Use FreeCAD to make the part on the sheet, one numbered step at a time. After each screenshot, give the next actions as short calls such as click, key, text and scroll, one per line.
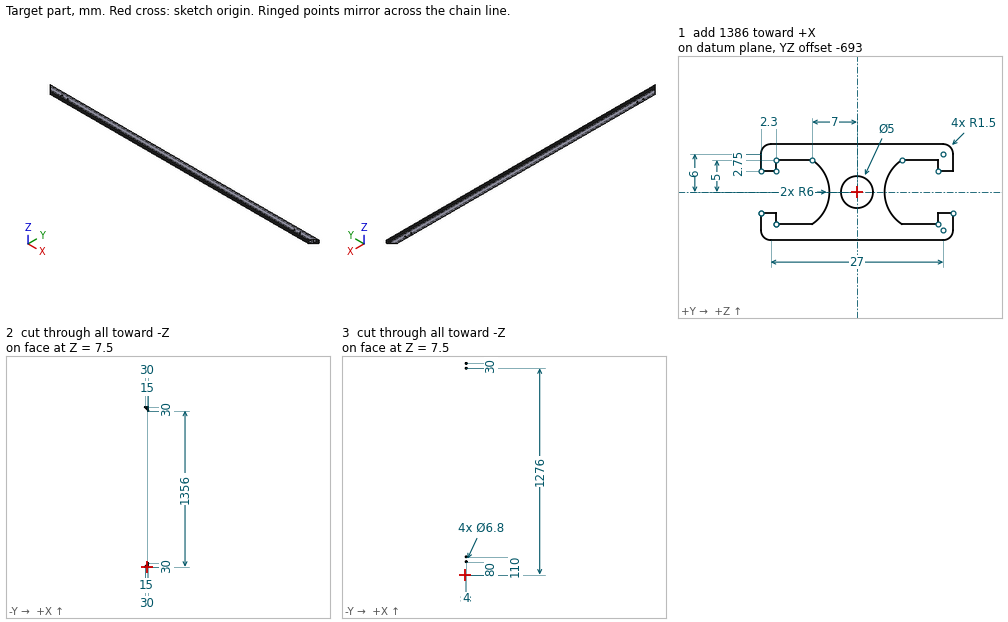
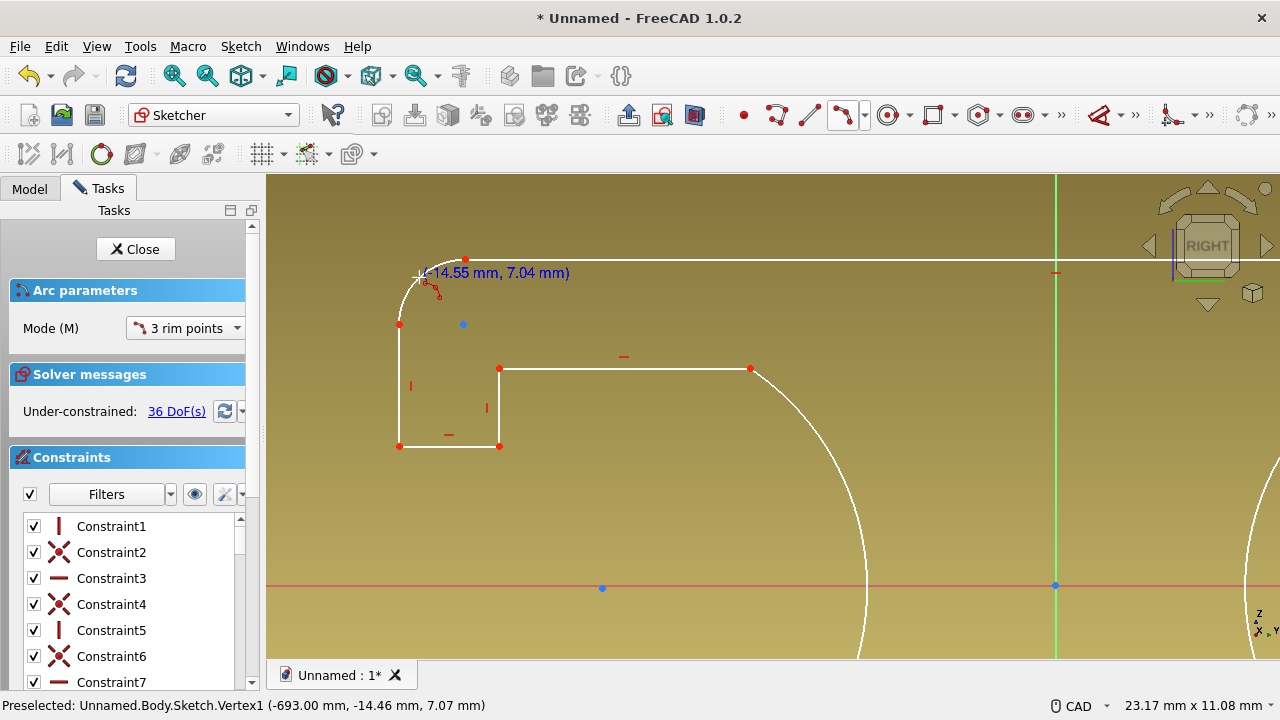
click(888, 116)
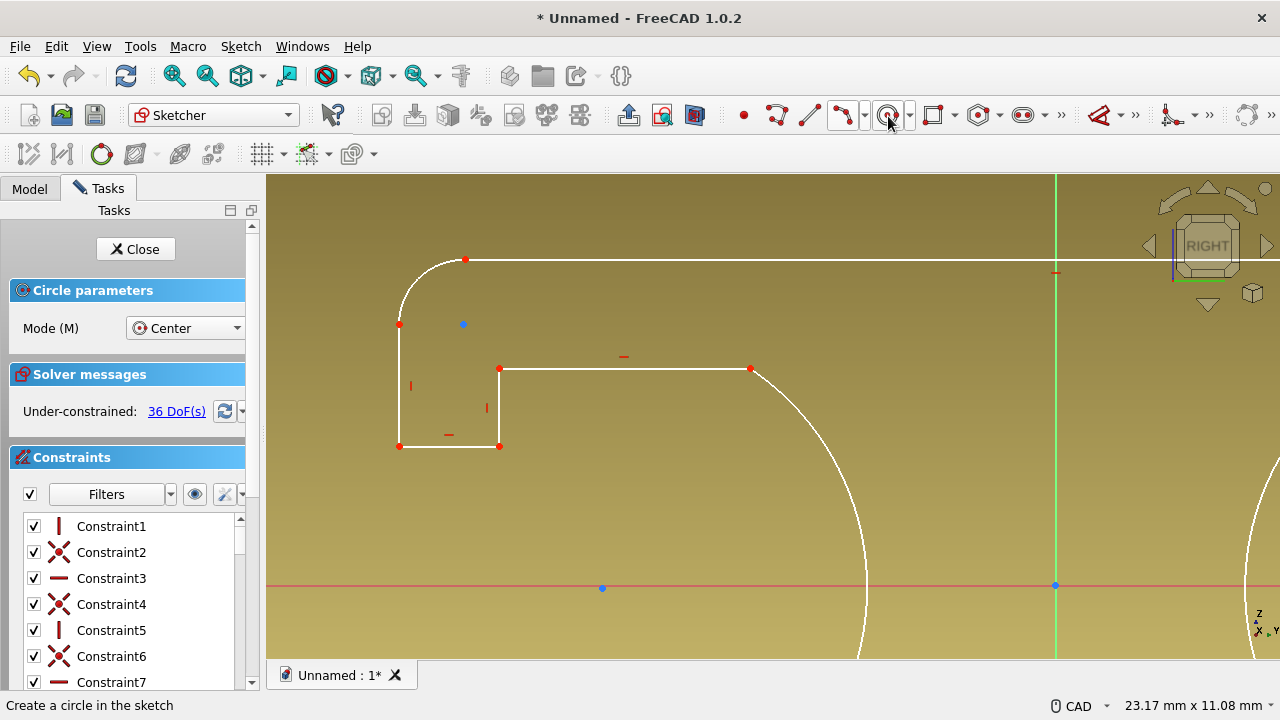
click(1056, 586)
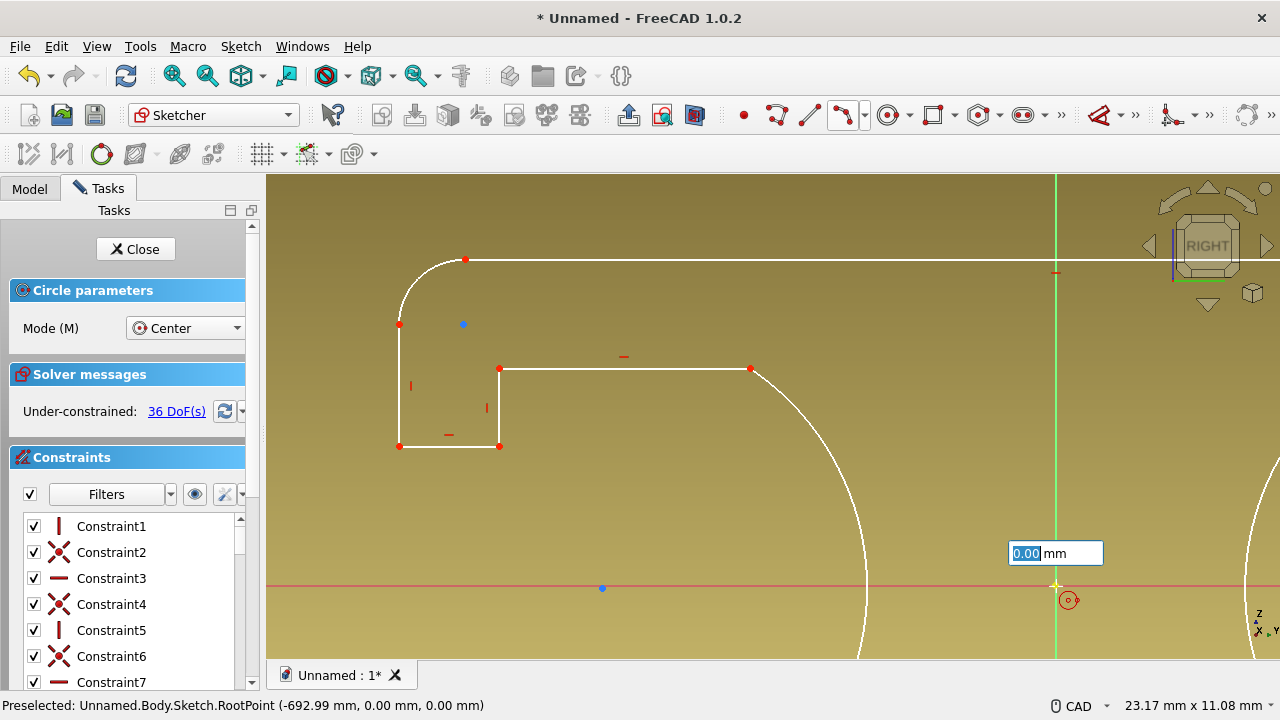
scroll(418, 278, down, 4)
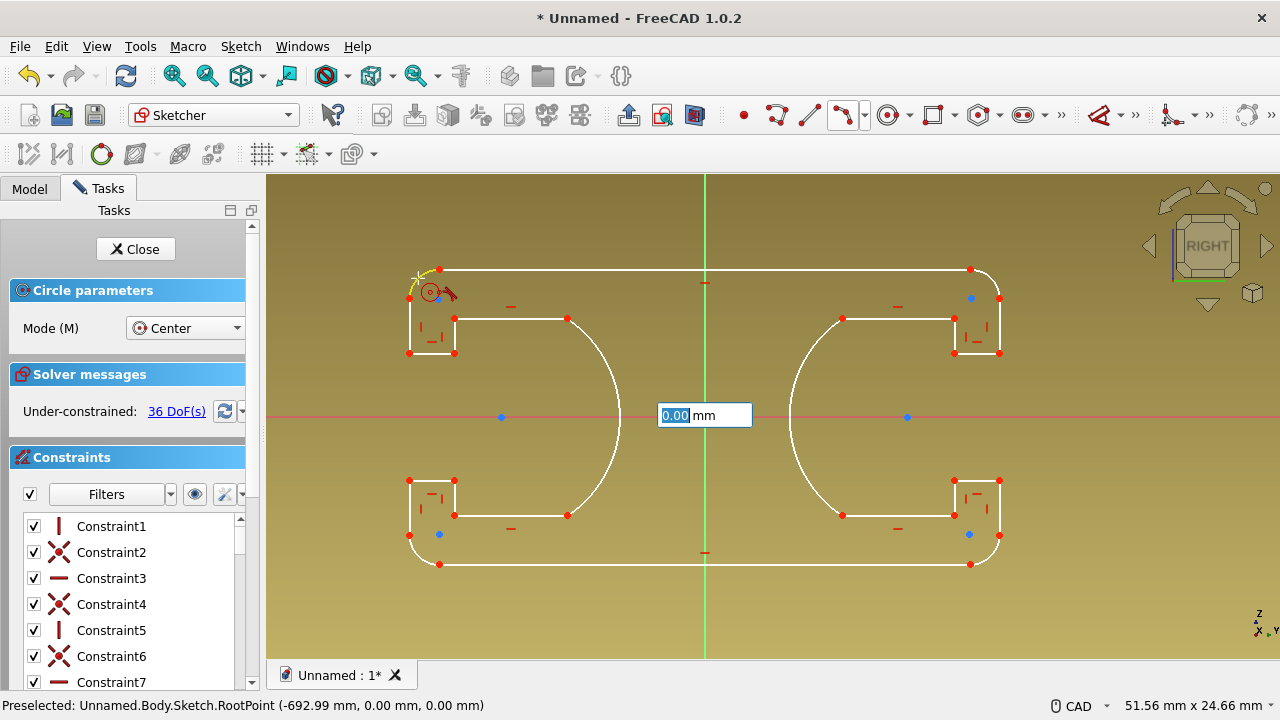
click(740, 382)
key(Escape)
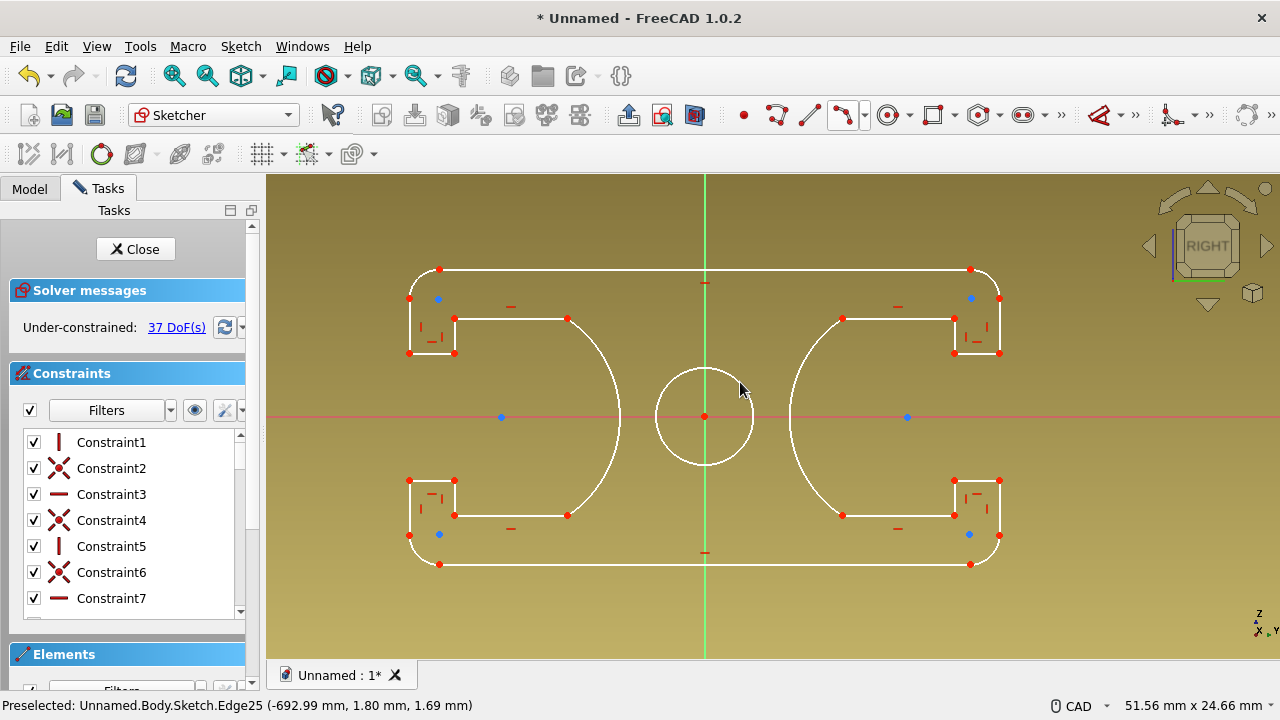
click(410, 315)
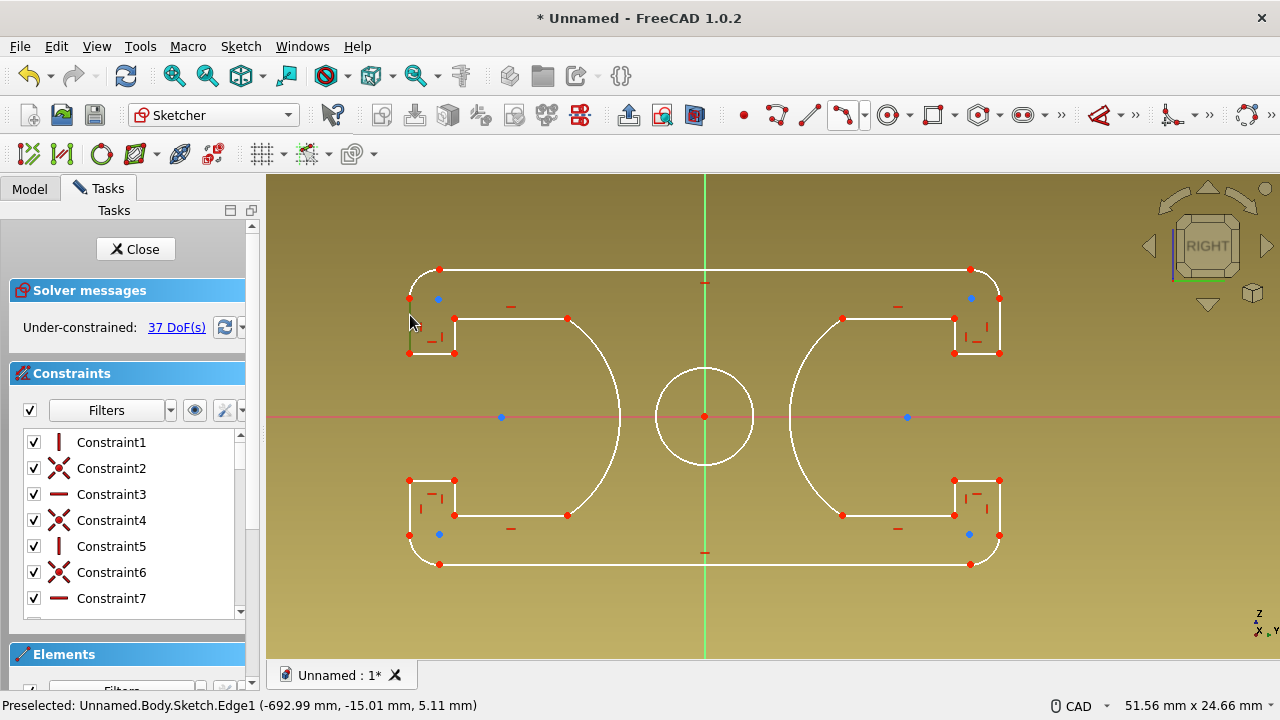
click(426, 273)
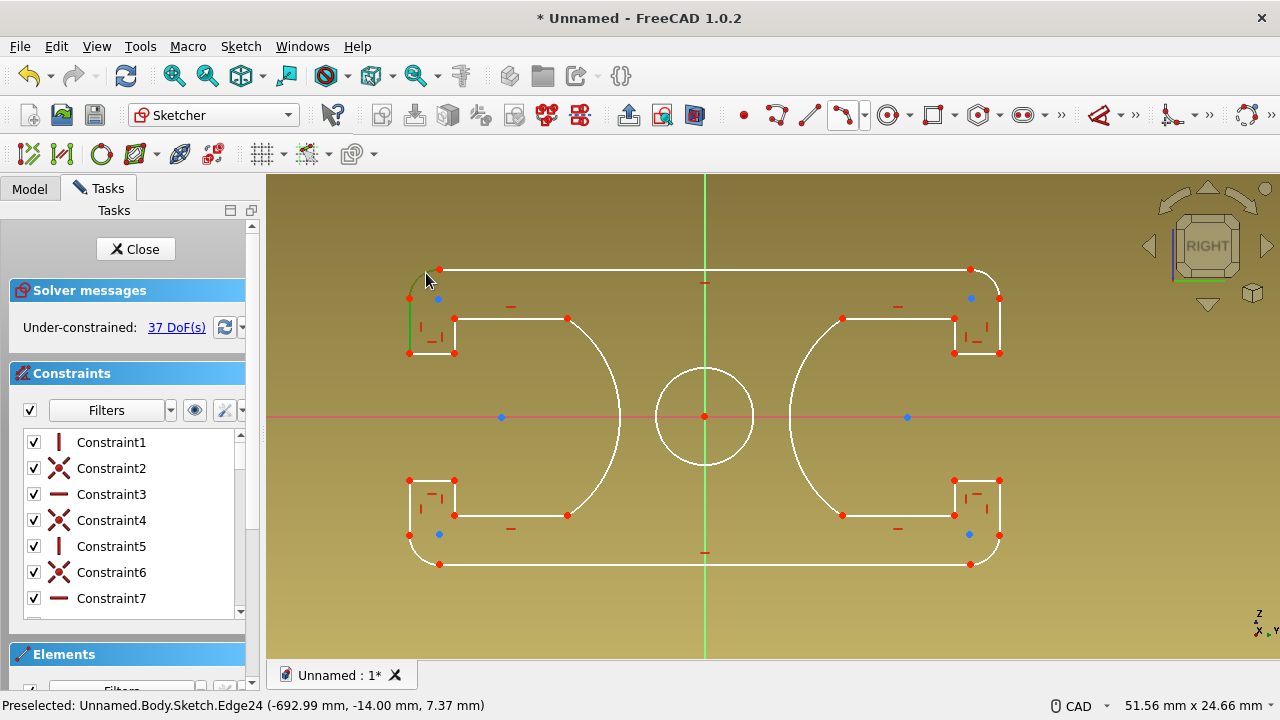
key(t)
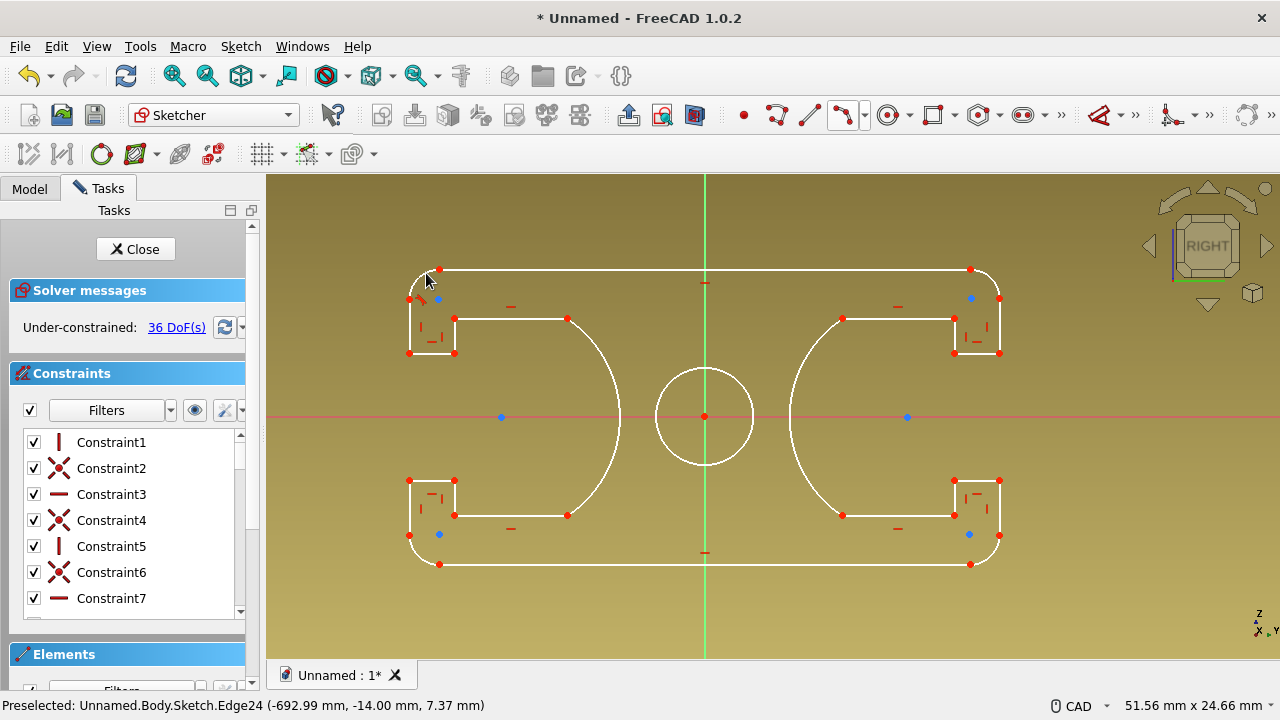
click(410, 497)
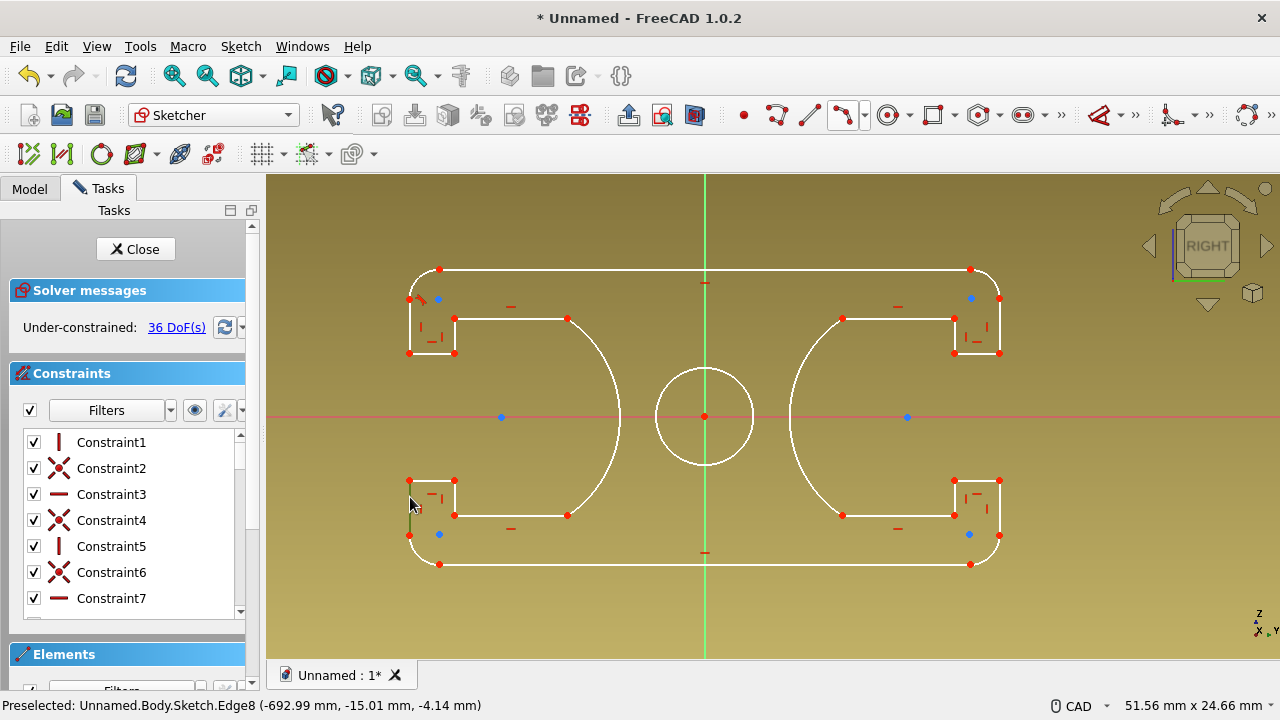
click(413, 549)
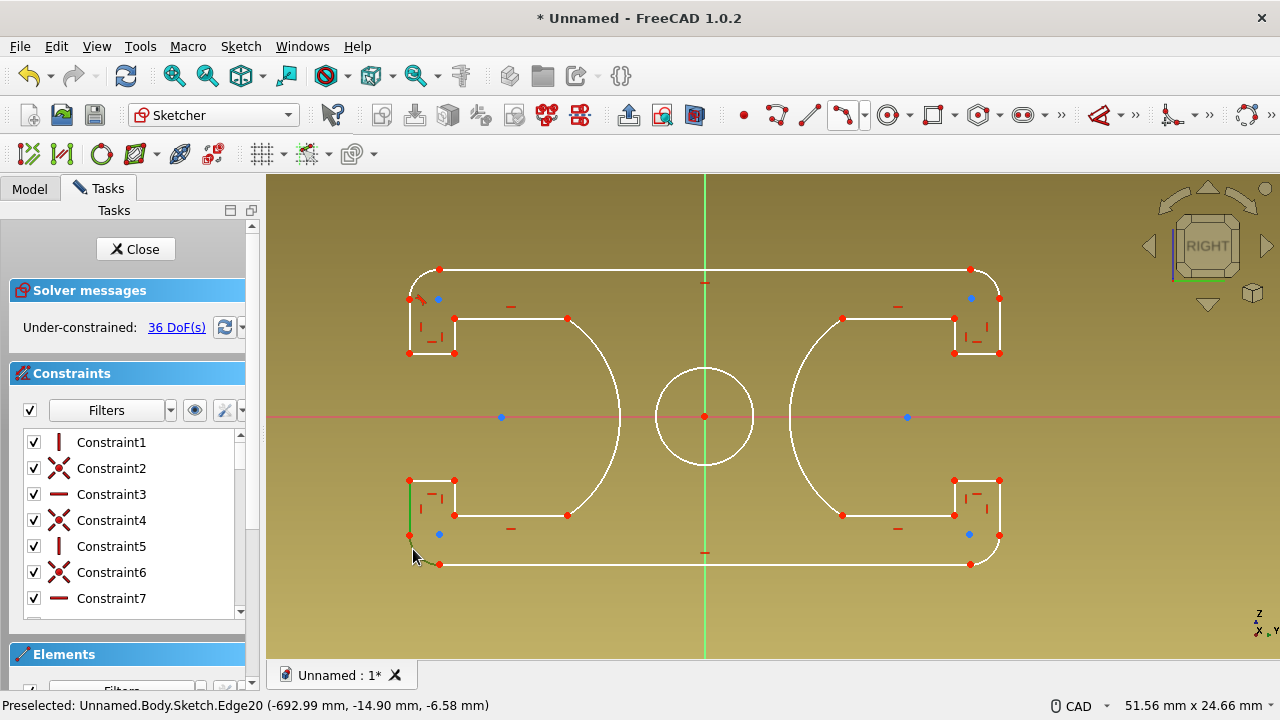
key(t)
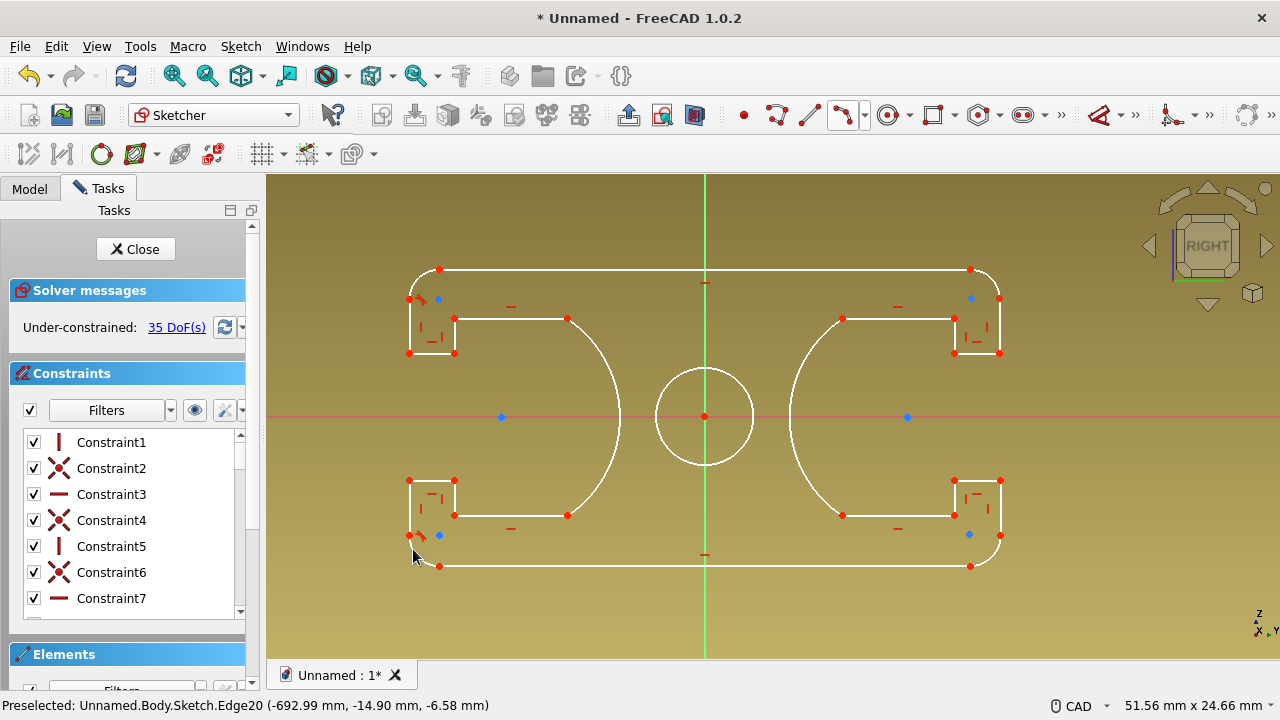
click(599, 566)